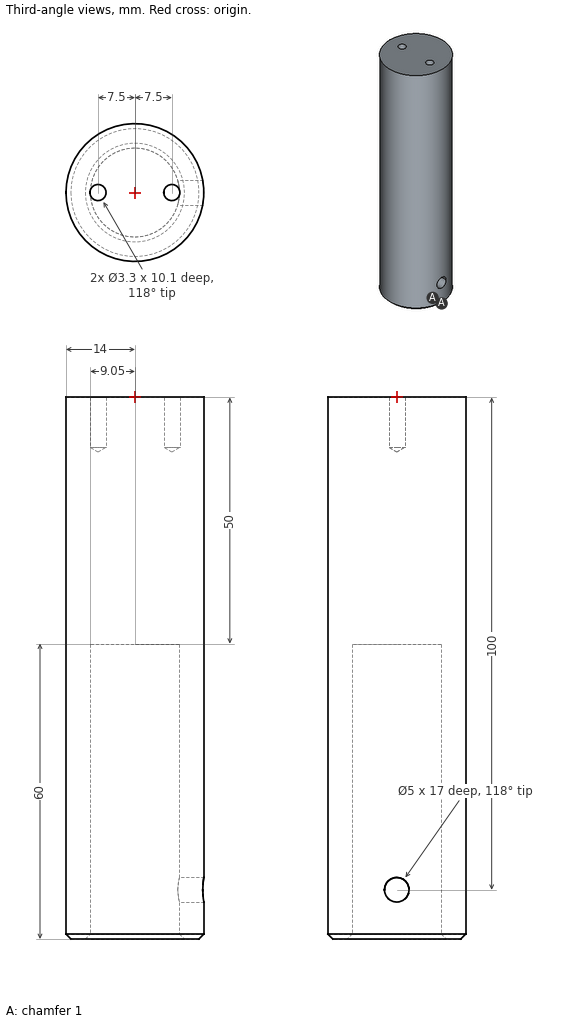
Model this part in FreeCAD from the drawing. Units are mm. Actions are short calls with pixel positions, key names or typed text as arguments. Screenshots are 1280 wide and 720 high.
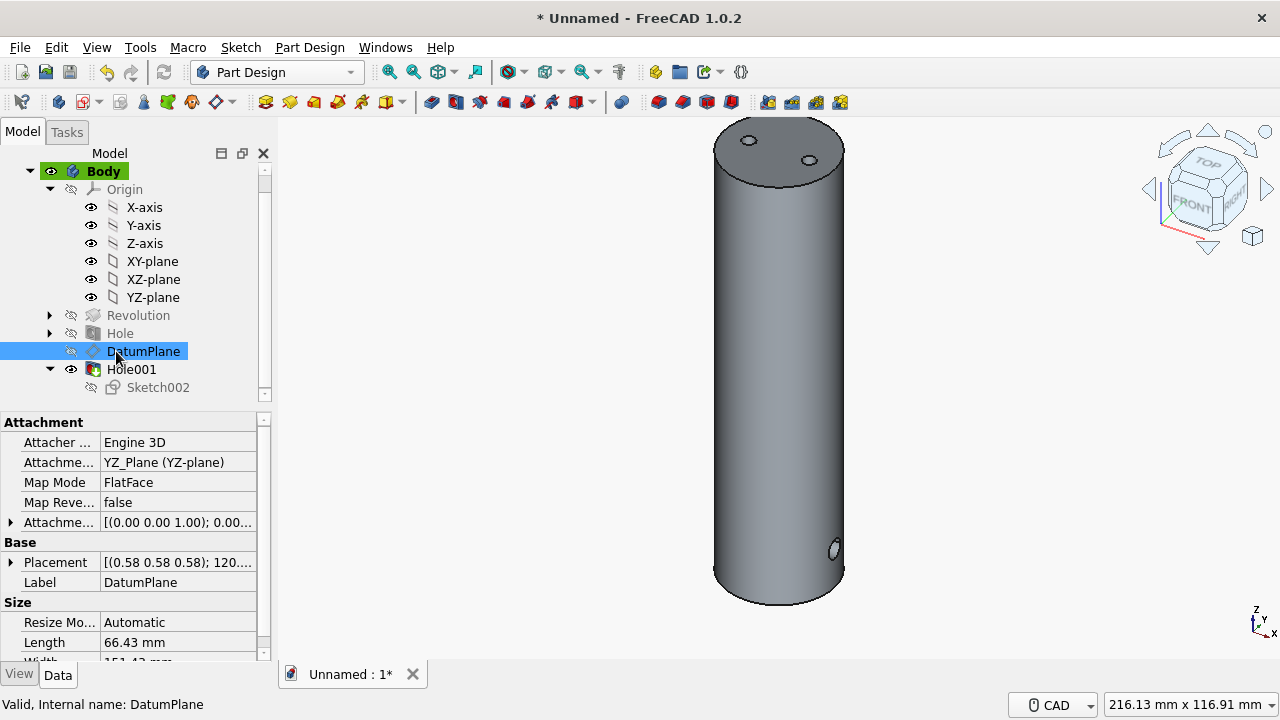
click(390, 72)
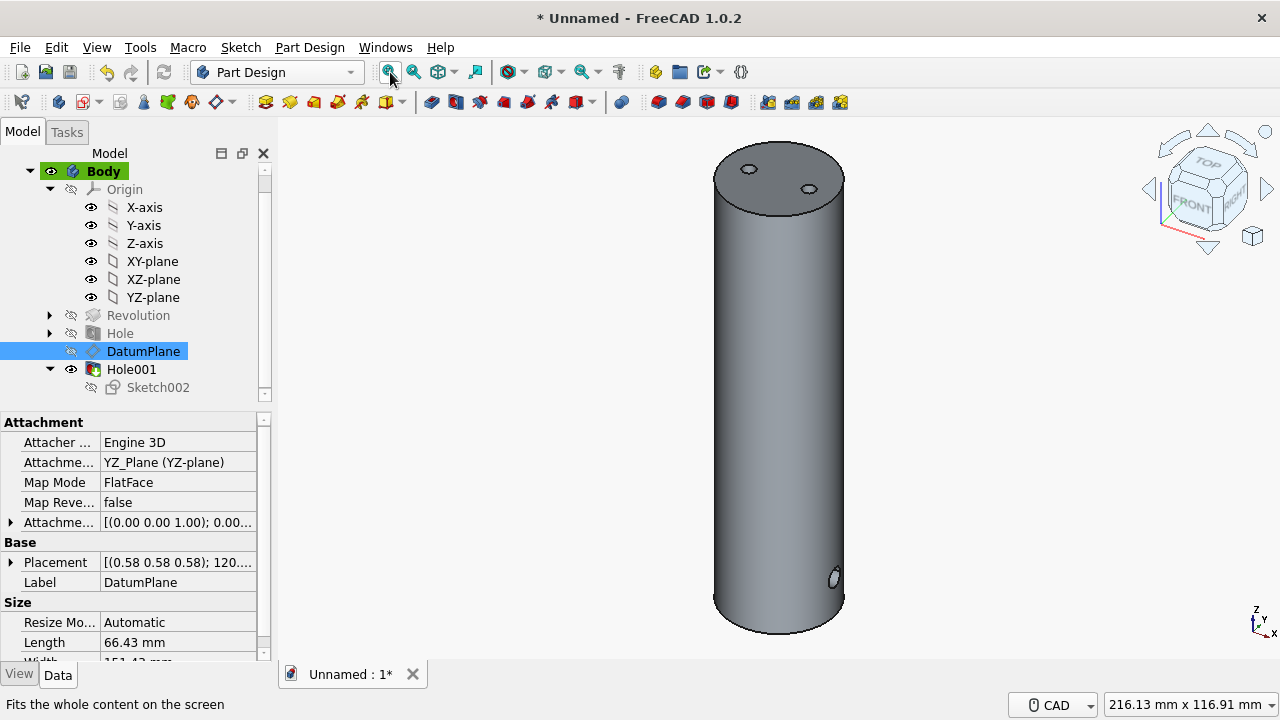
key(0)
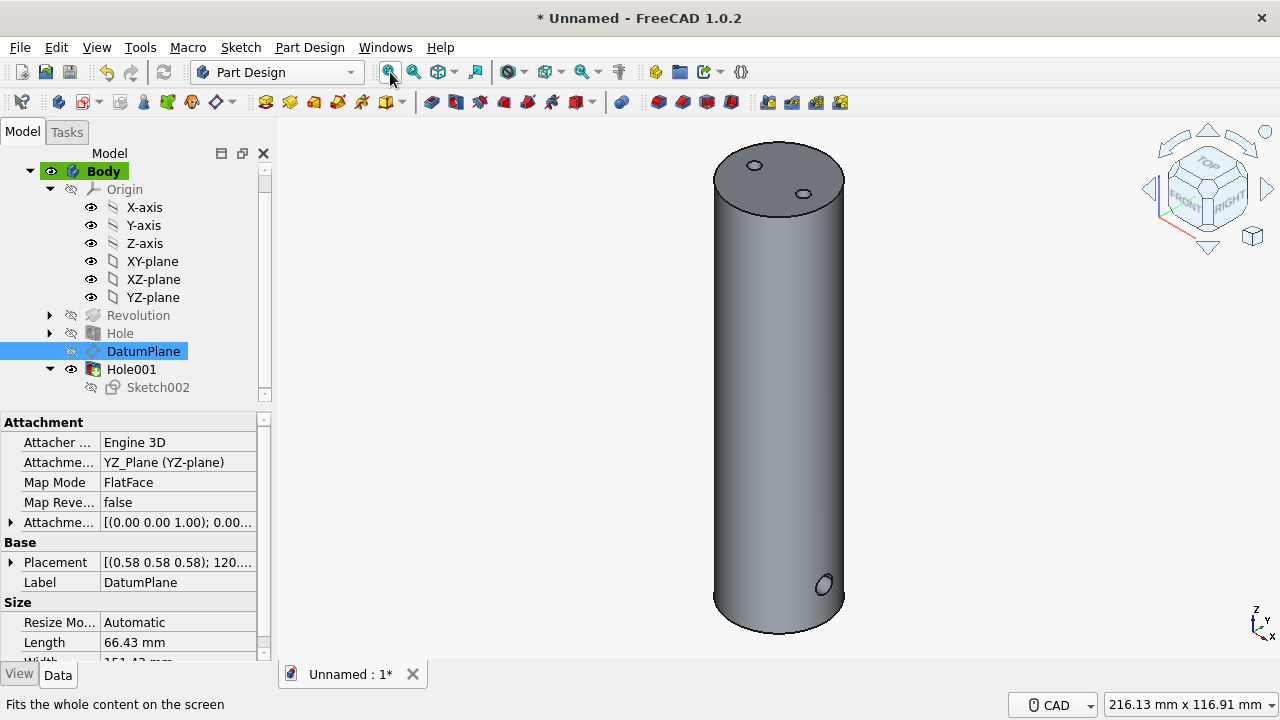
key(2)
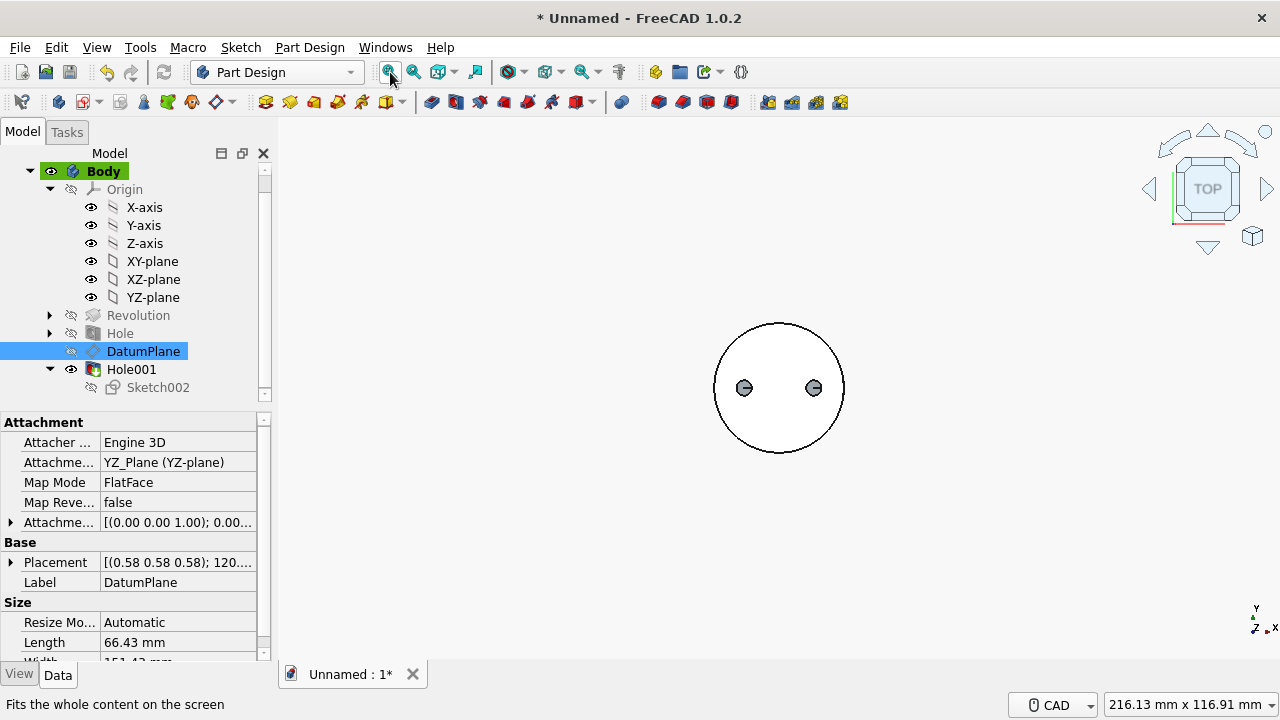
click(390, 72)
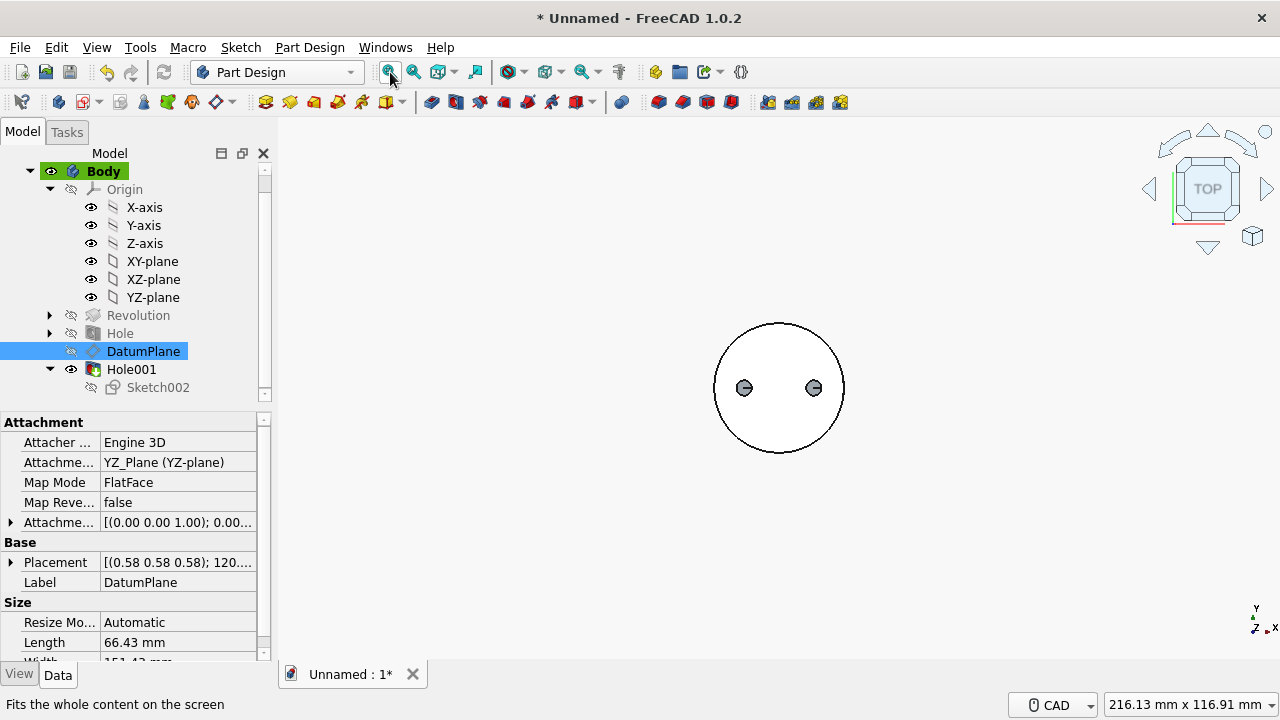
key(1)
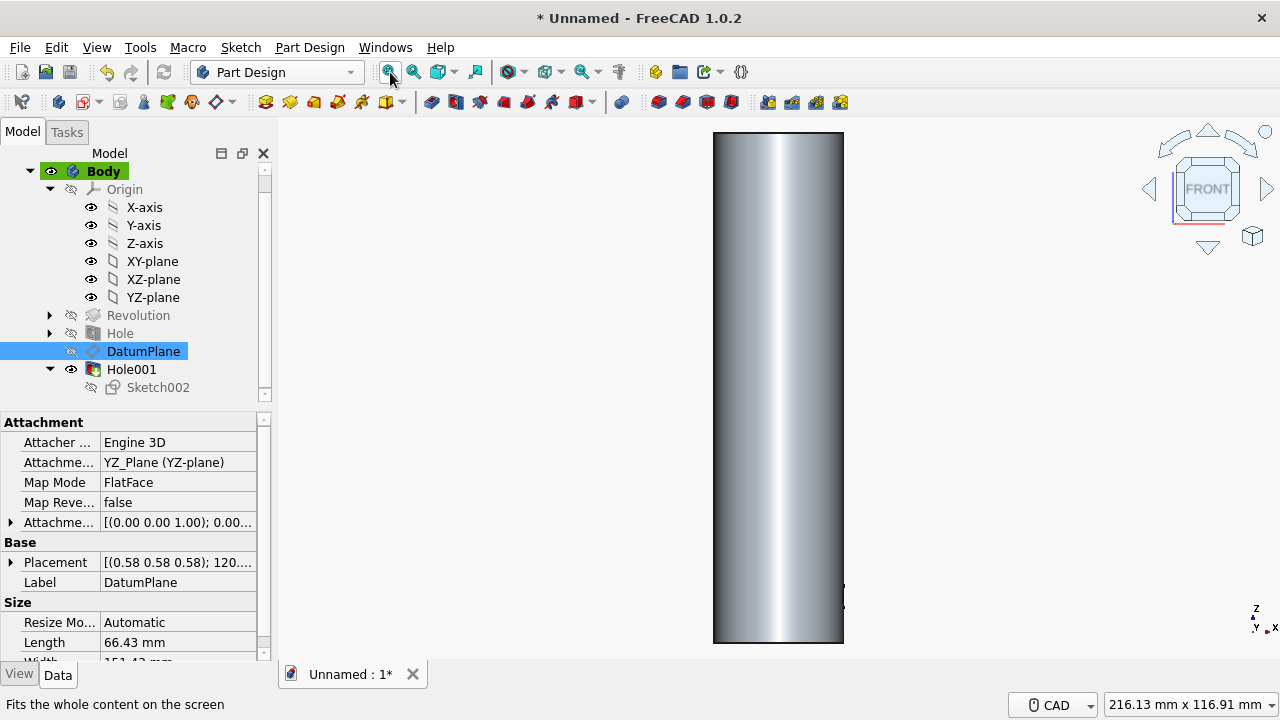
key(3)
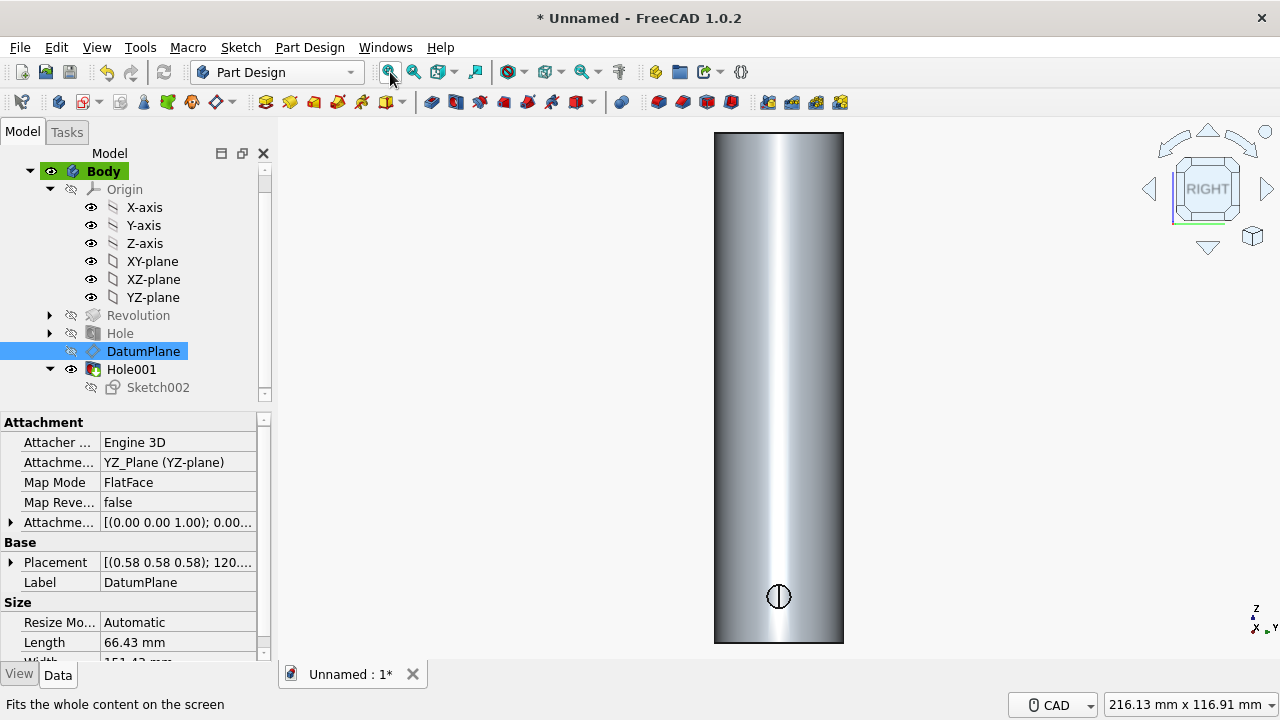
key(5)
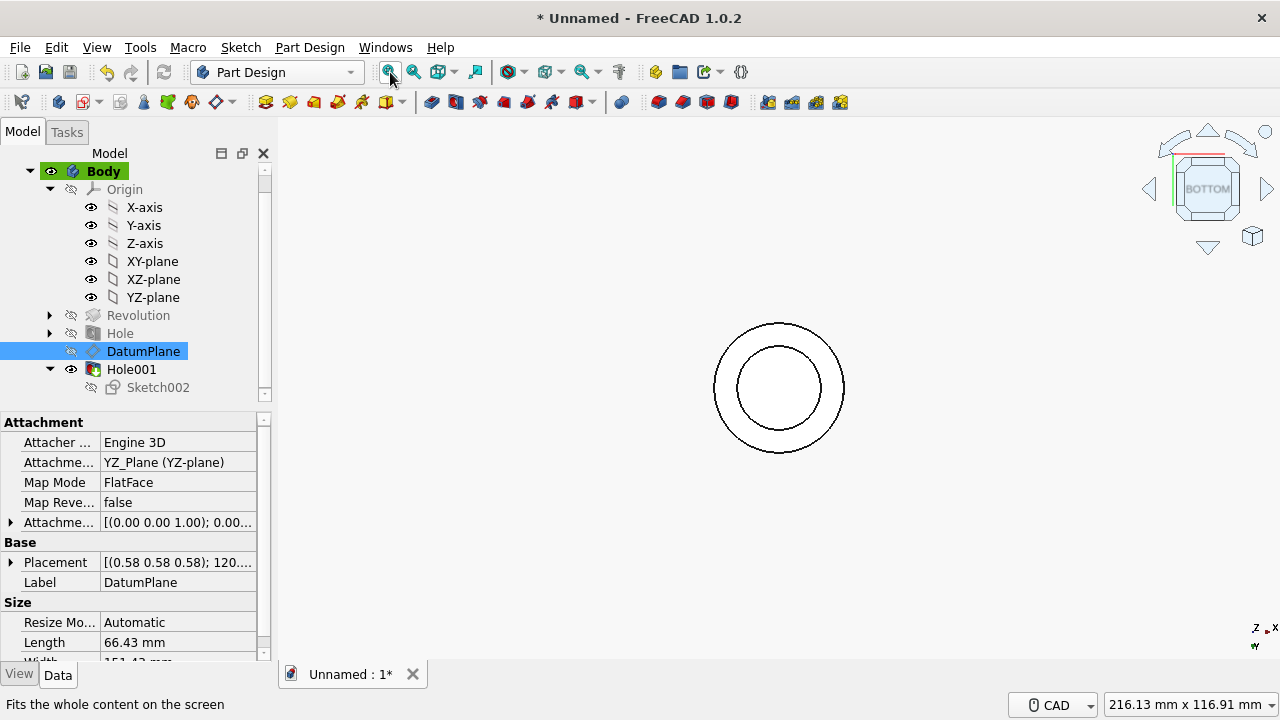
click(390, 72)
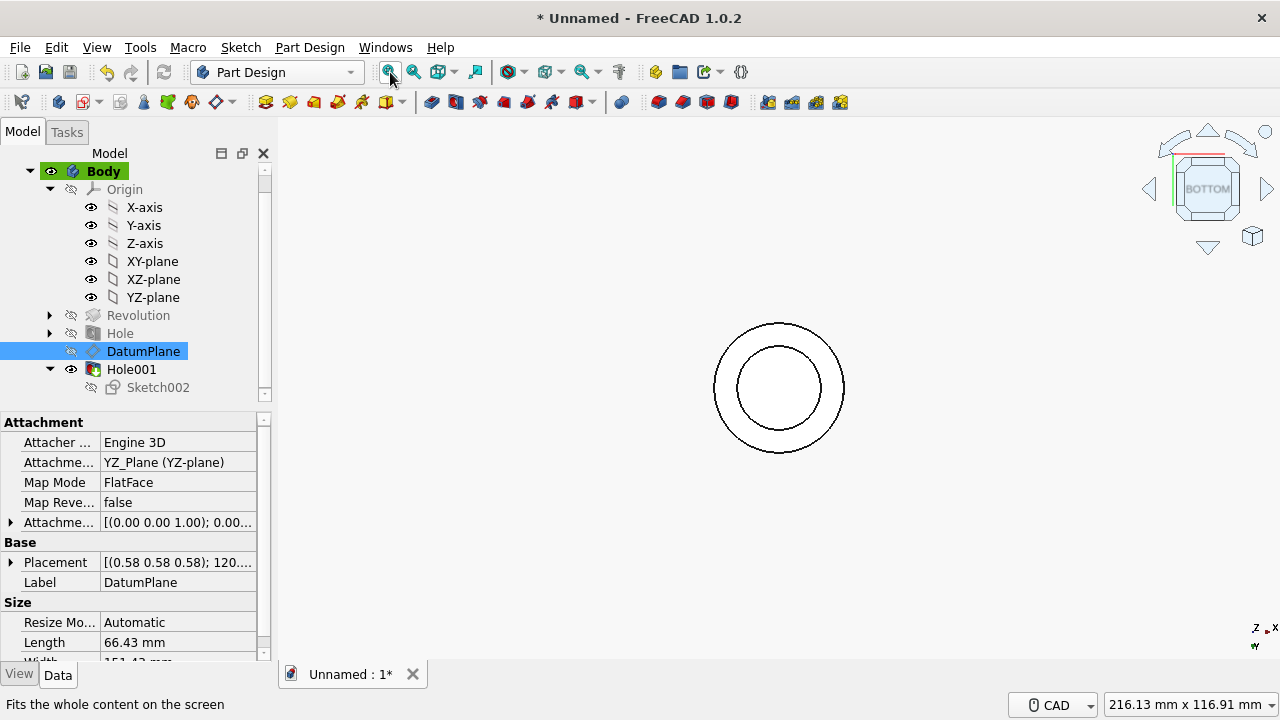
click(844, 387)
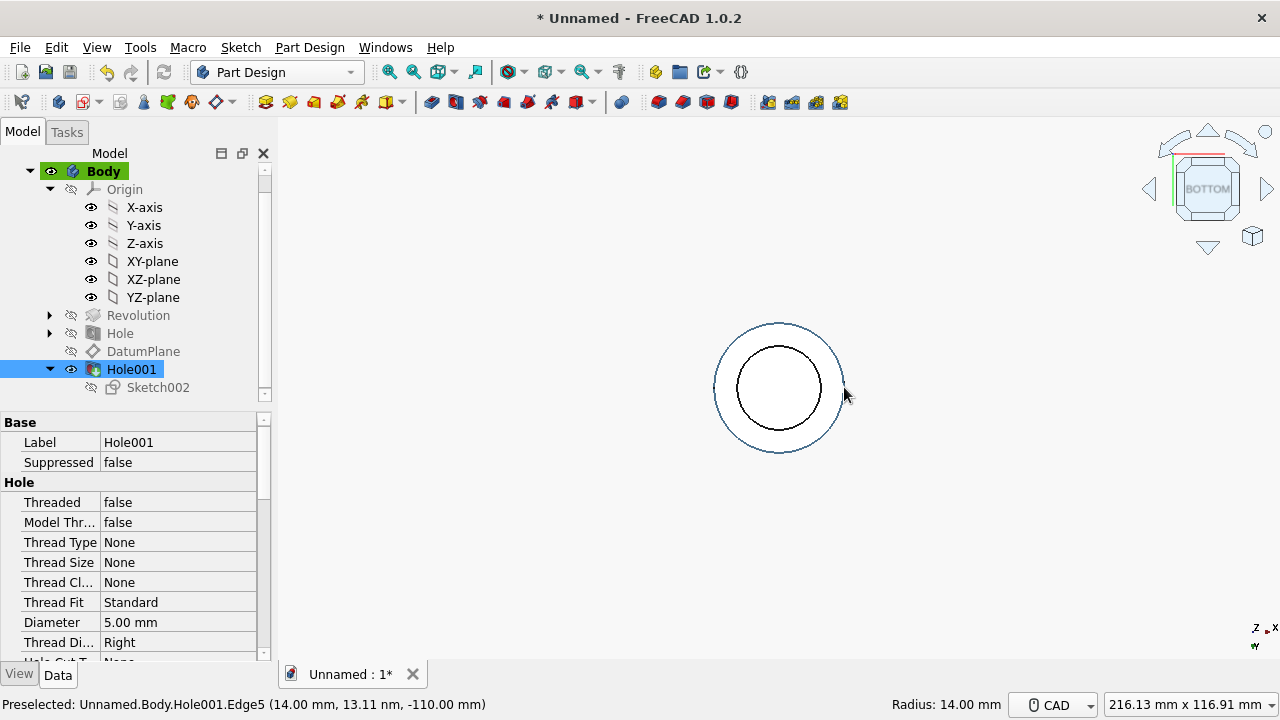
click(821, 387, ctrl)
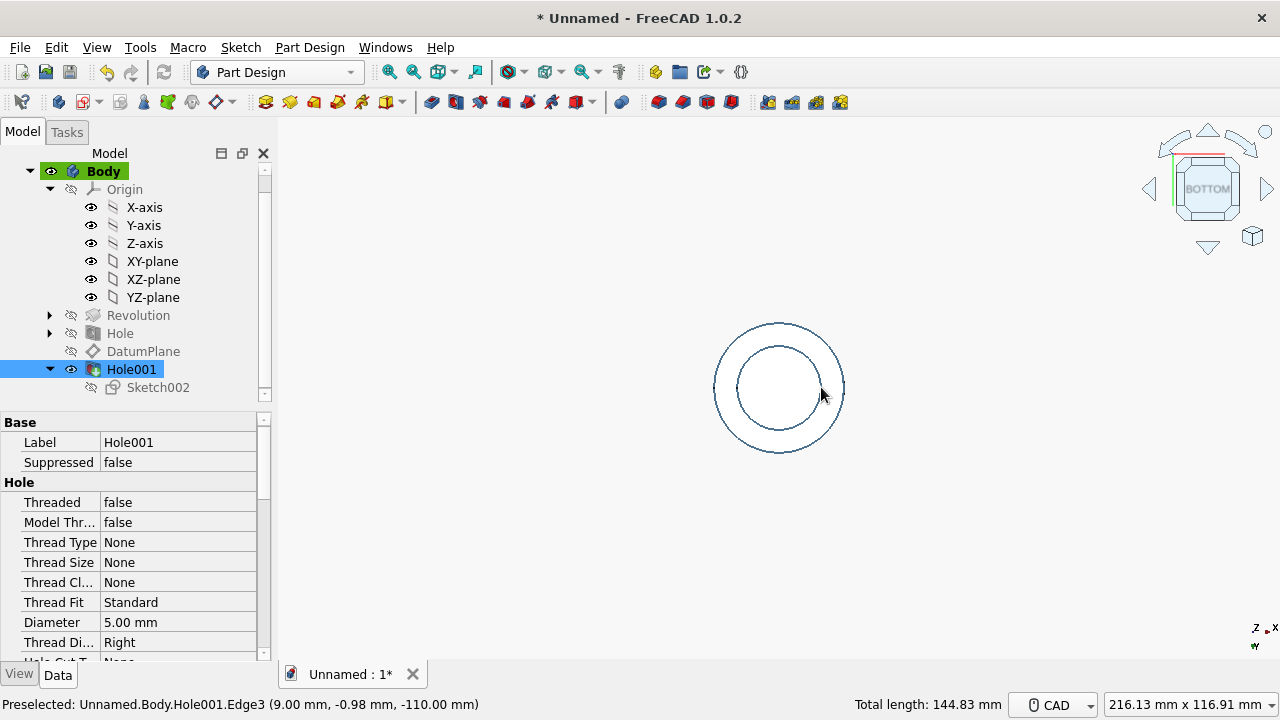
click(684, 102)